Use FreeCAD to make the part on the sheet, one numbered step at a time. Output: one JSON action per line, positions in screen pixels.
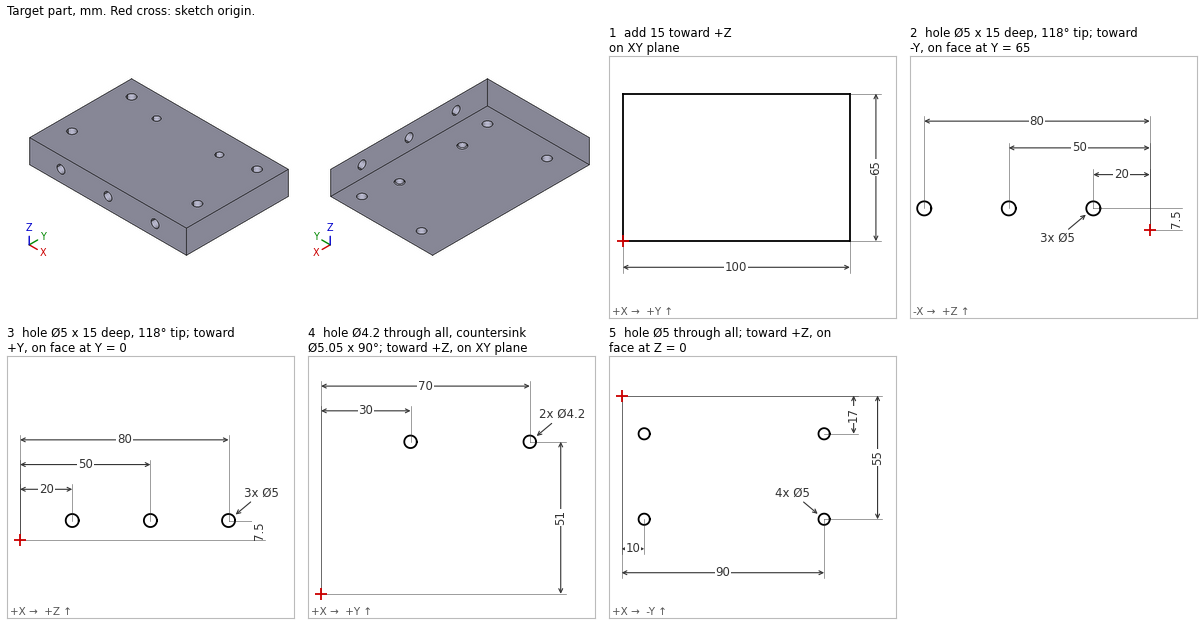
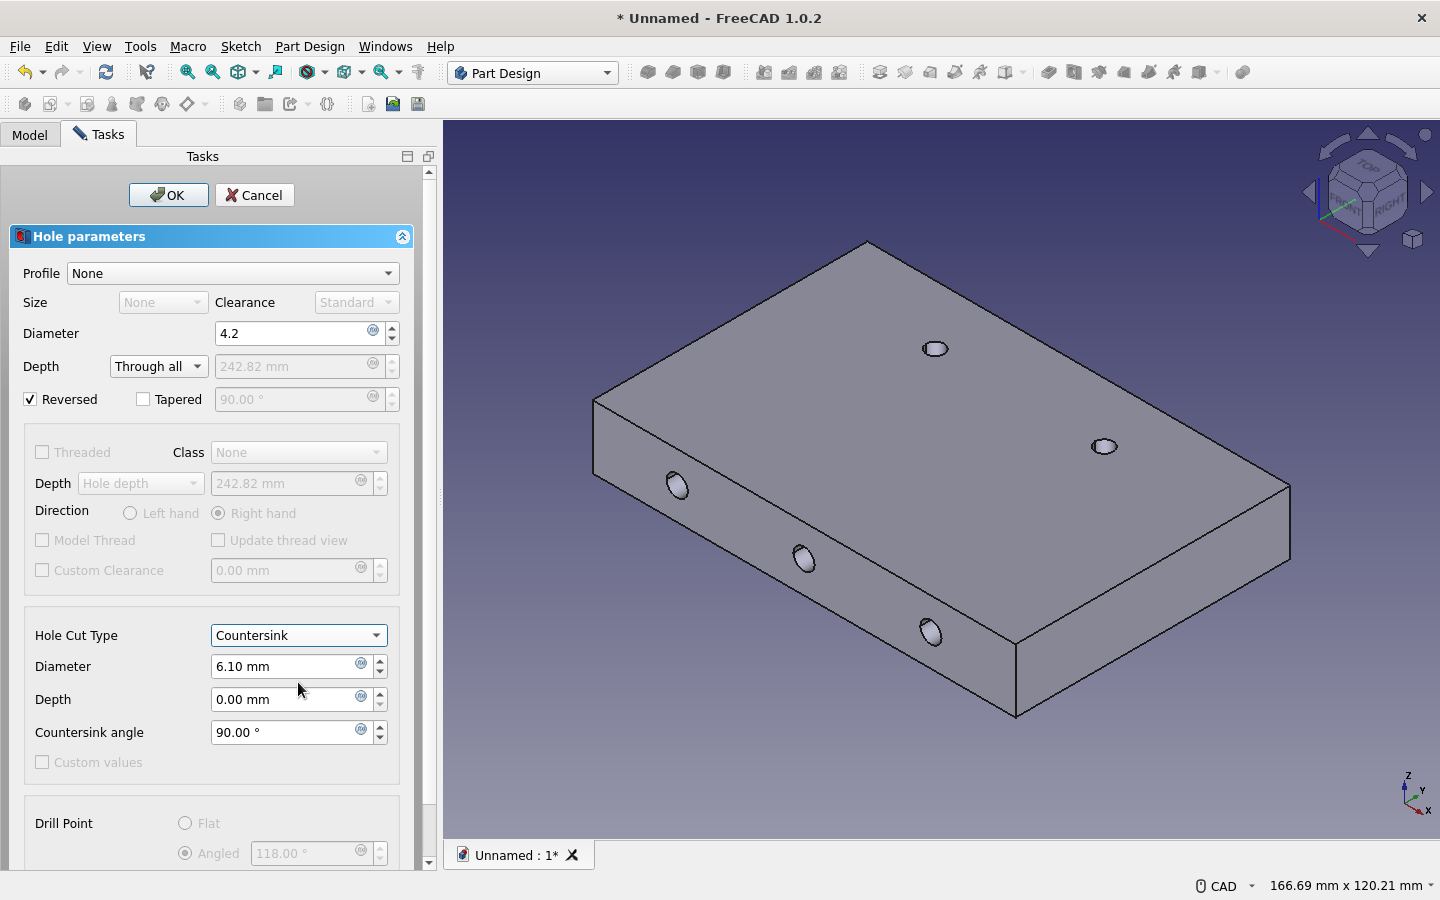
{"action": "triple_click", "coordinate": [292, 666]}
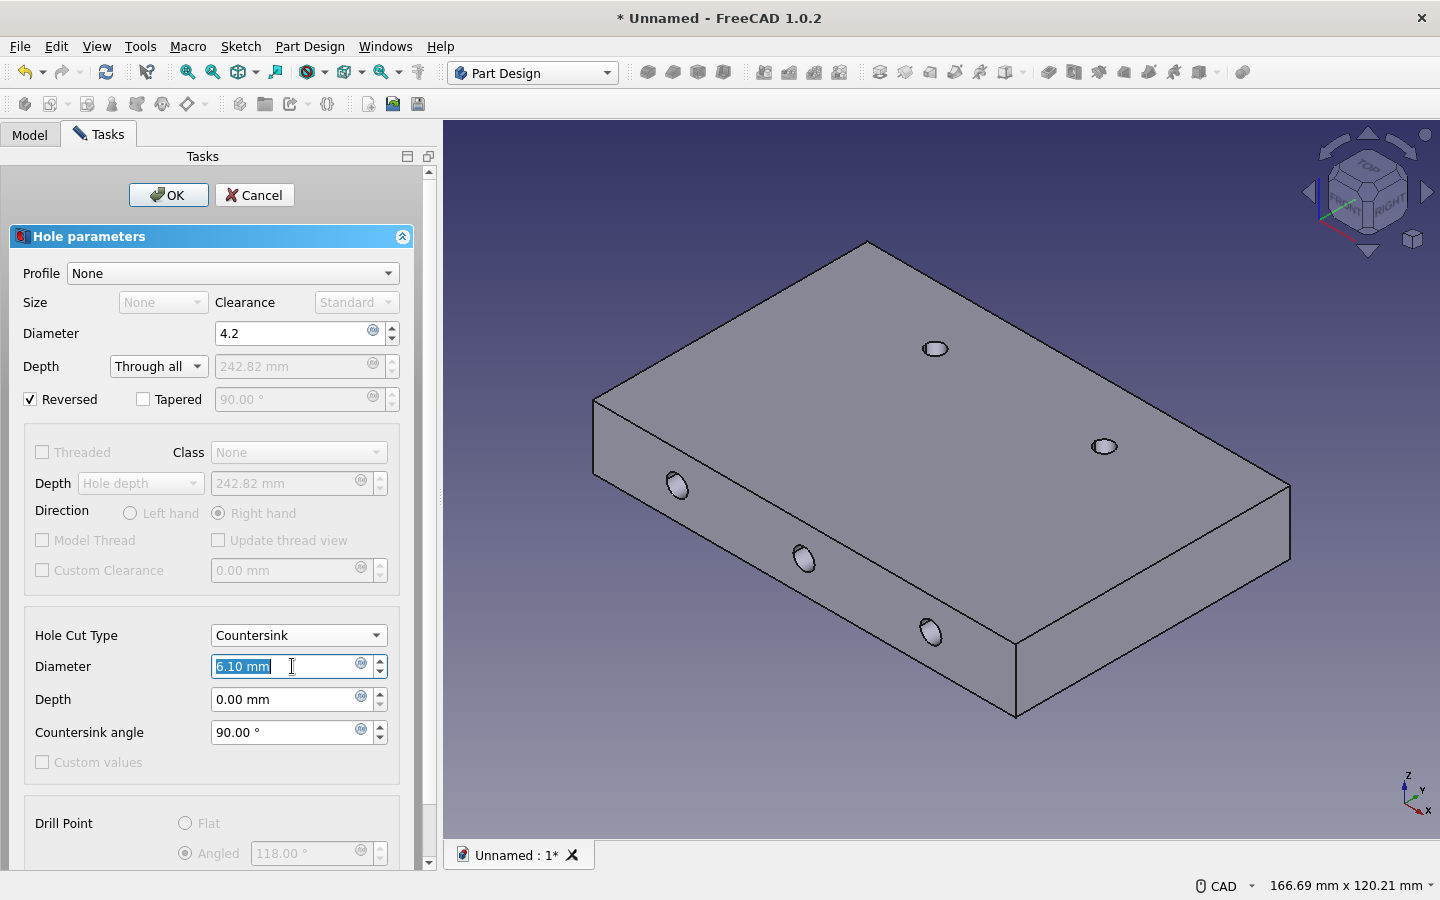
{"action": "type", "text": "5.05"}
{"action": "key", "text": "Tab"}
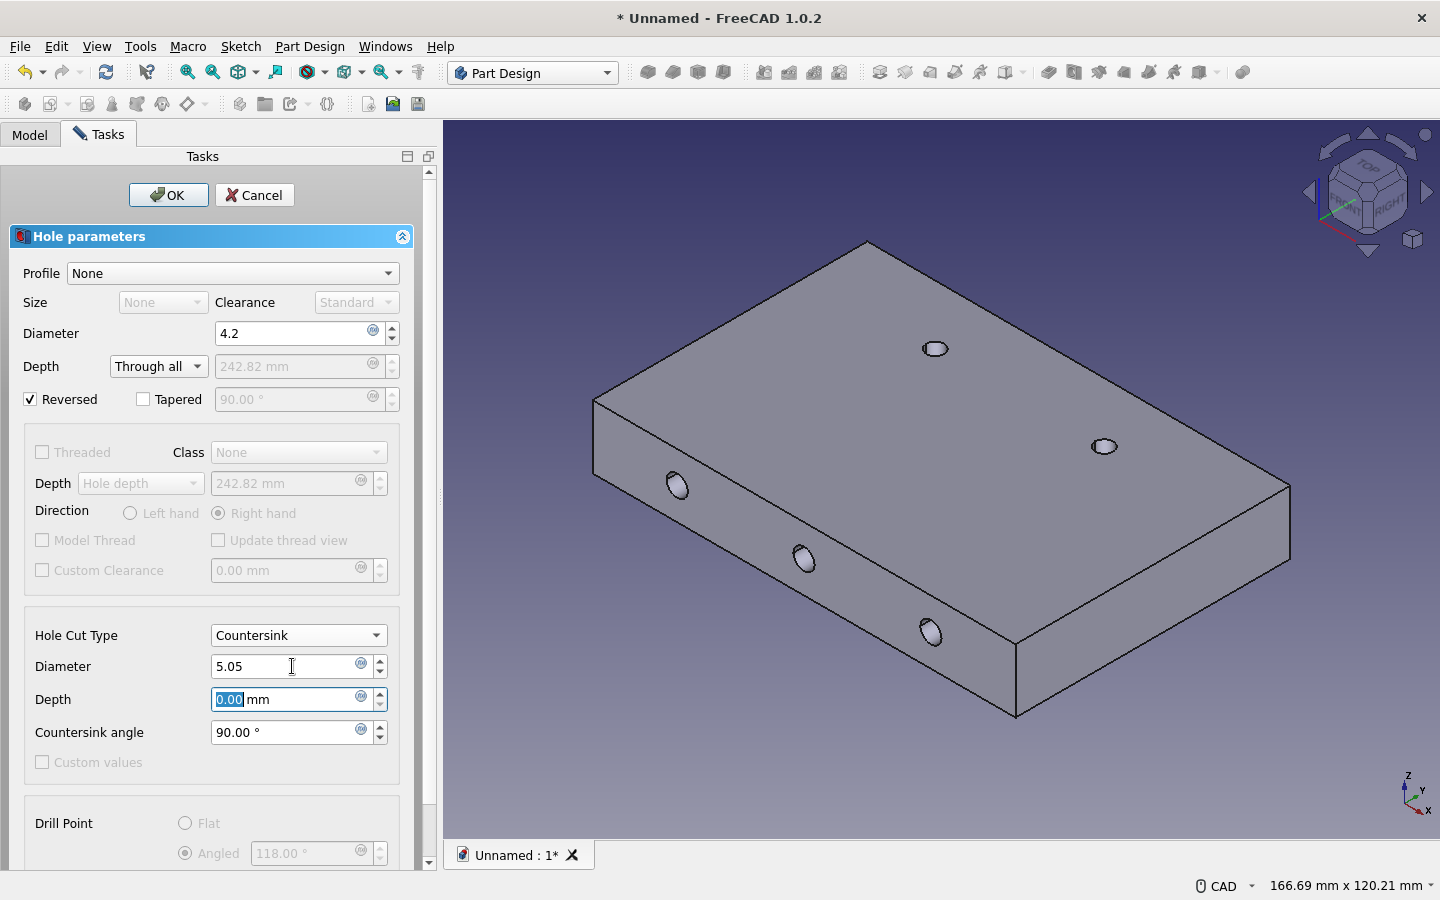
{"action": "left_click", "coordinate": [169, 195]}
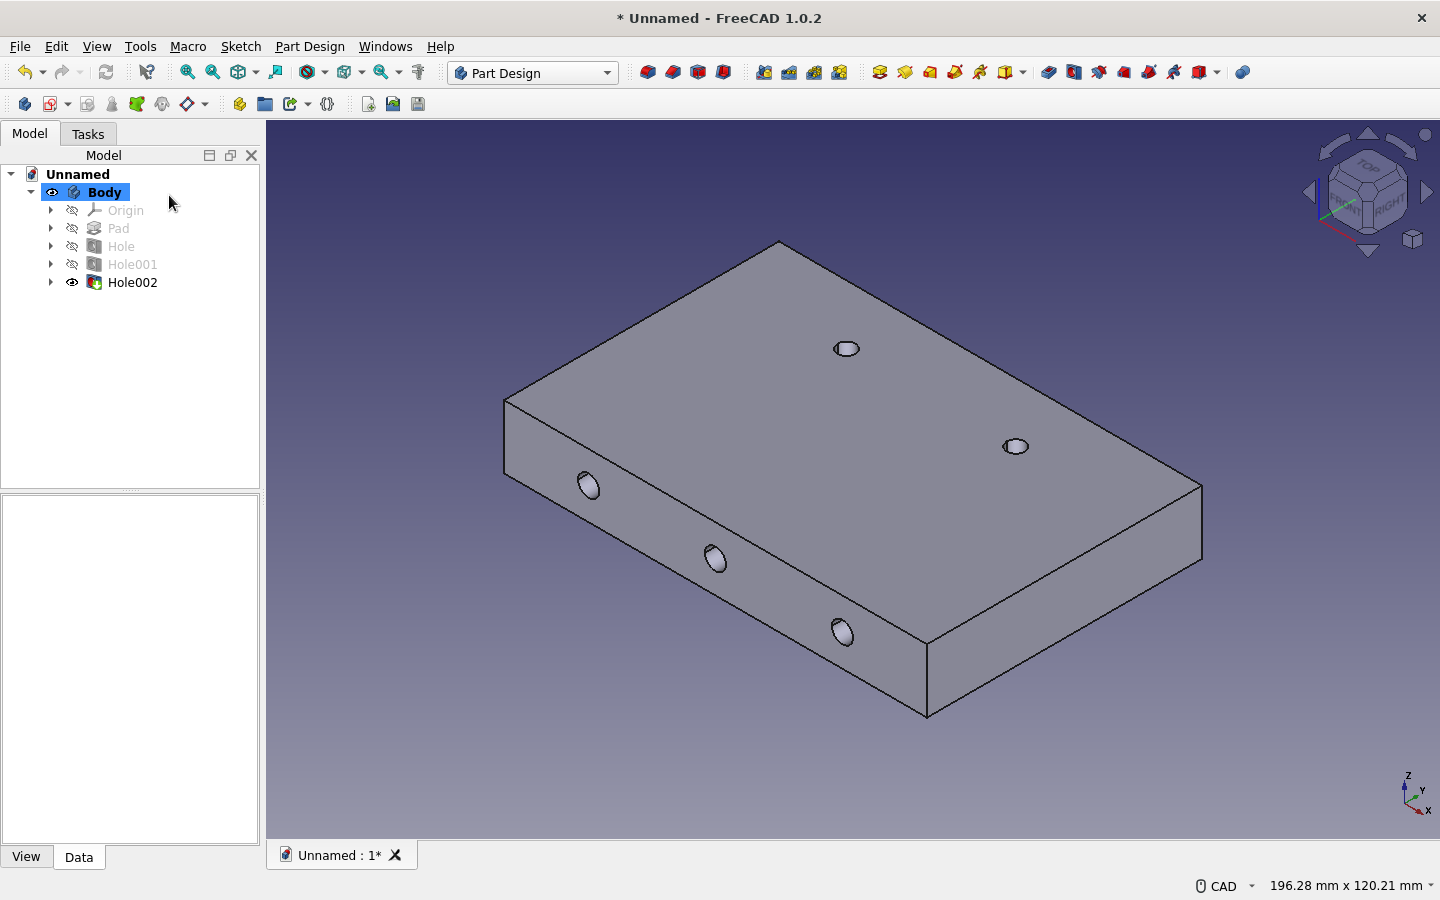
{"action": "key", "text": "5"}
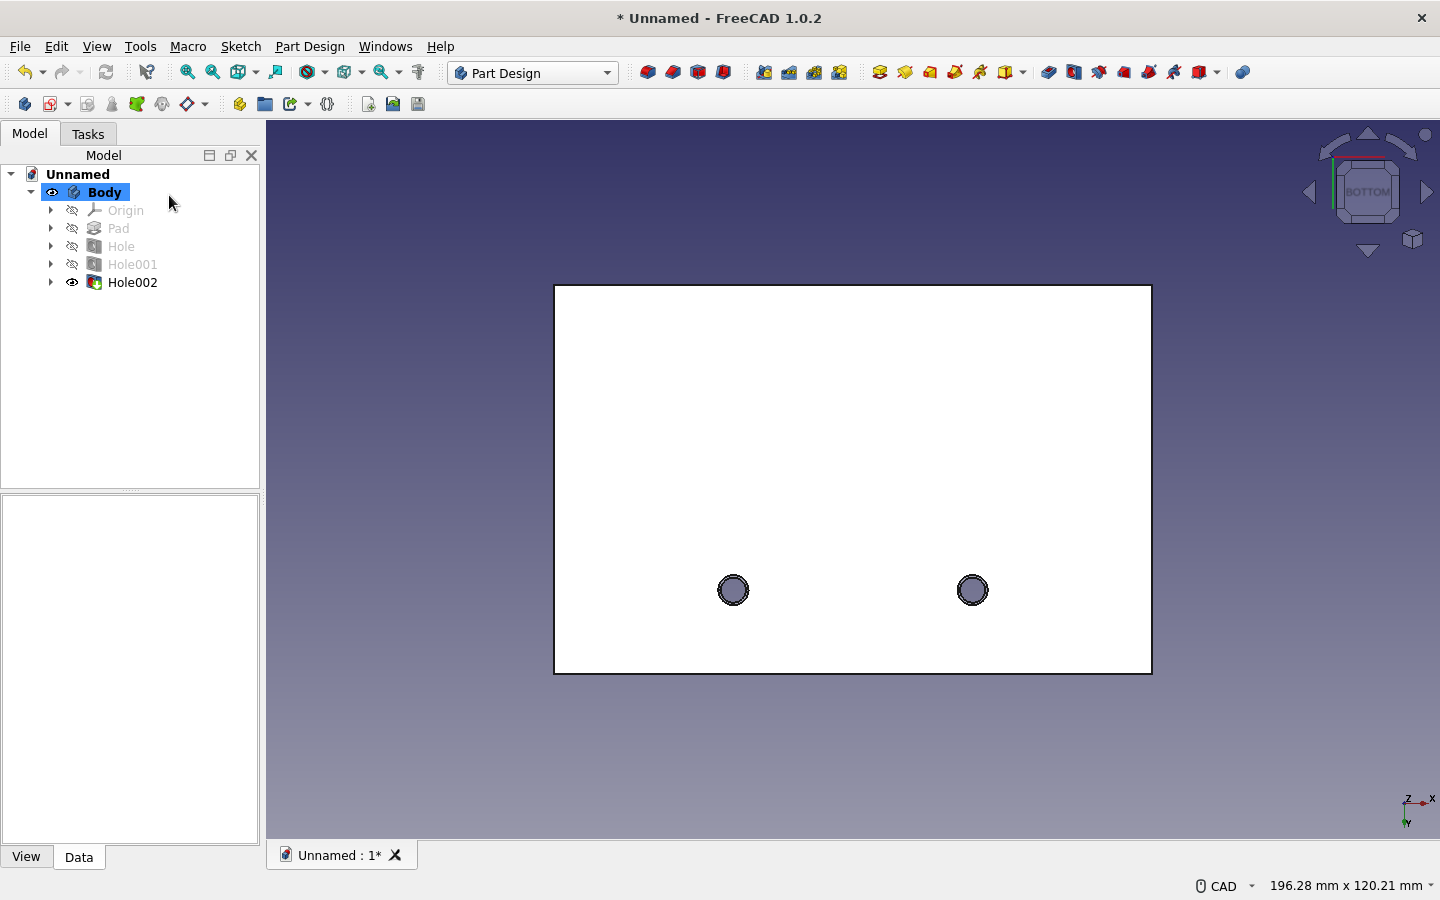
{"action": "left_click", "coordinate": [853, 479]}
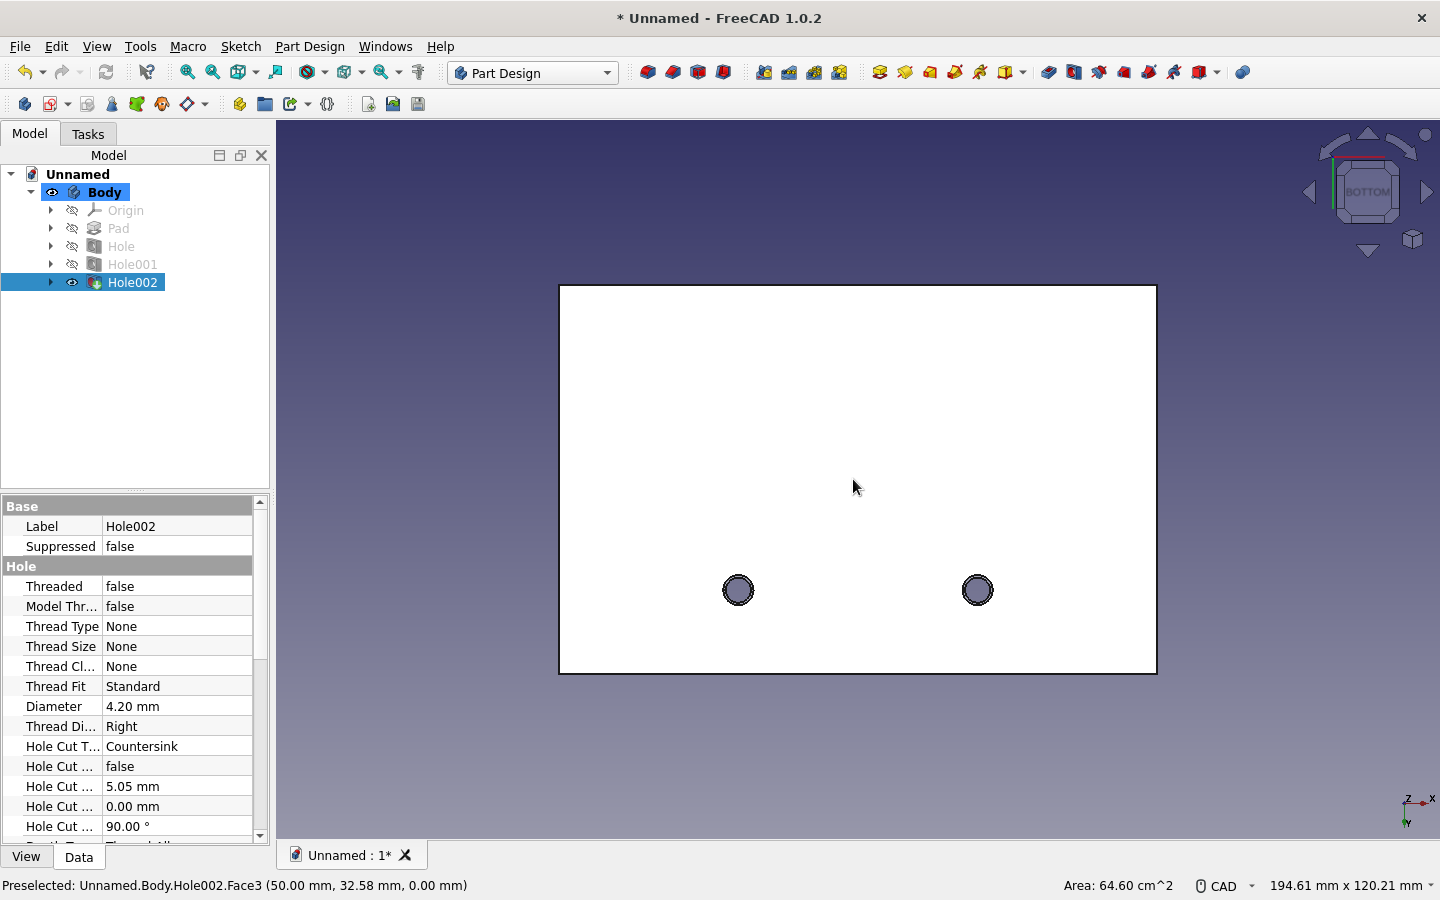
{"action": "left_click", "coordinate": [50, 104]}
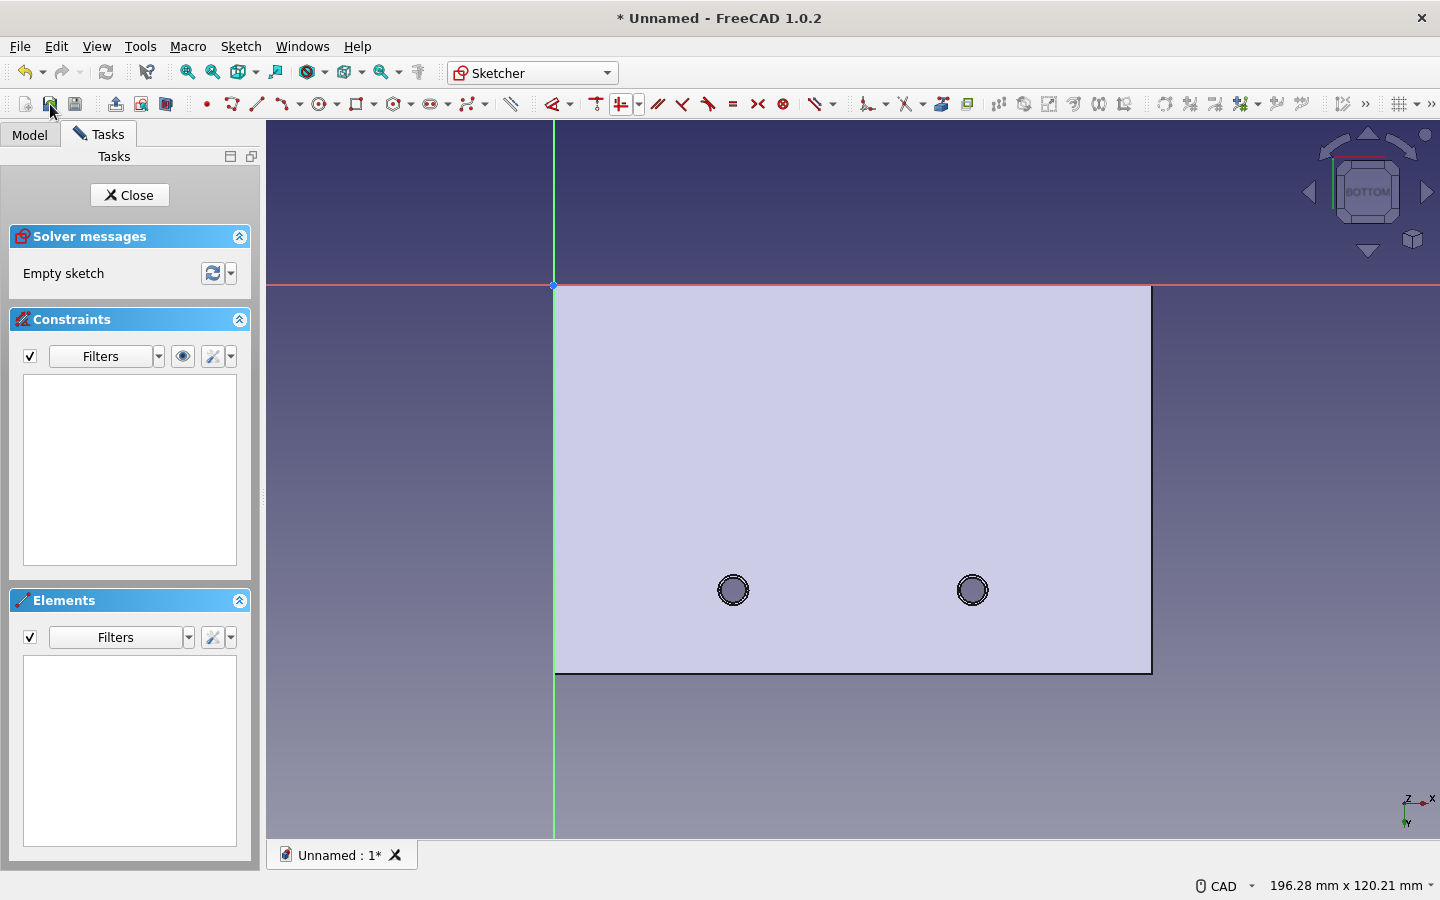
{"action": "key", "text": "g c"}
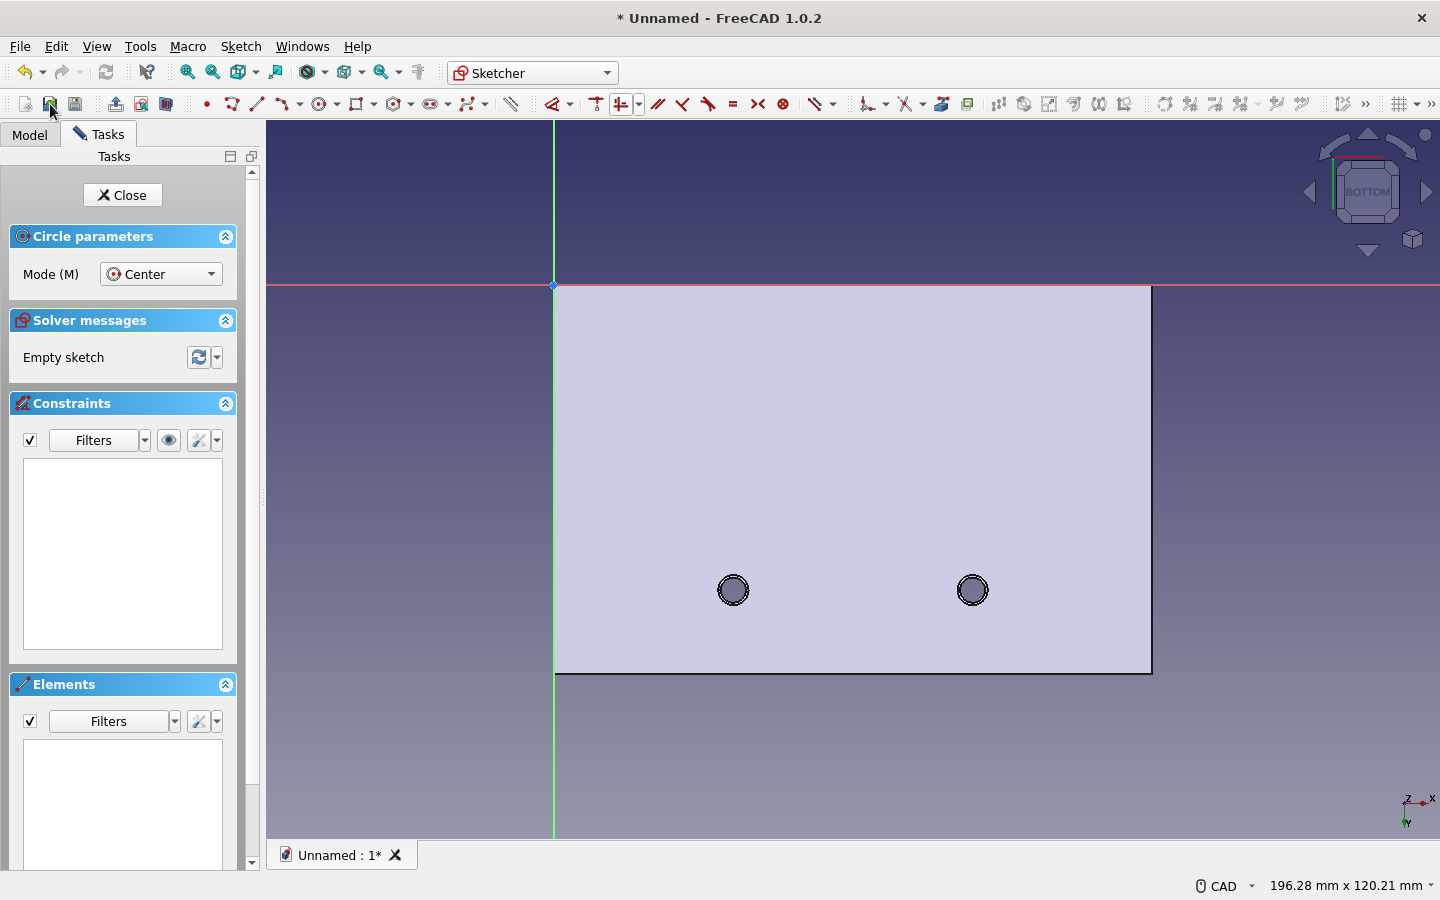
{"action": "scroll", "coordinate": [1092, 614], "scroll_direction": "up", "scroll_amount": 3}